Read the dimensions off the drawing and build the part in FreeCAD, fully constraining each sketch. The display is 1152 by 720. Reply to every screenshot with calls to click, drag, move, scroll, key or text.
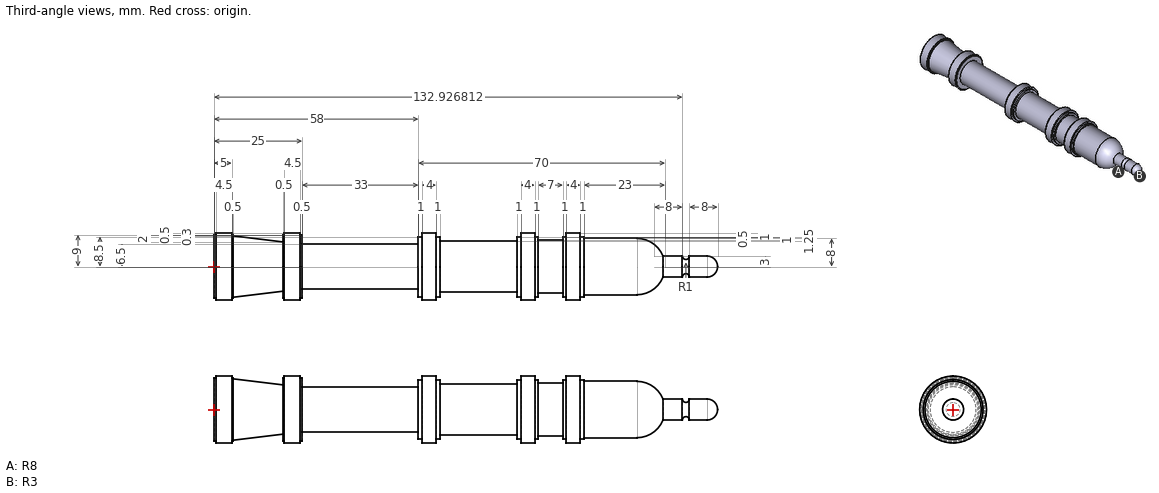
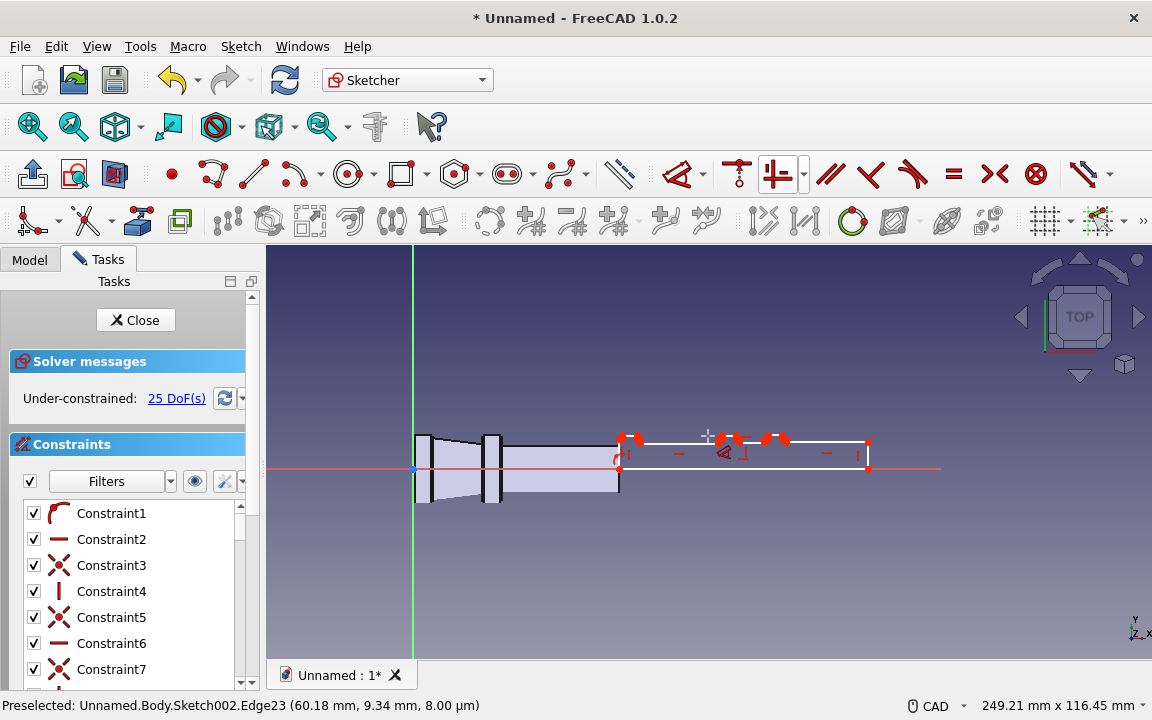
scroll(868, 461, up, 3)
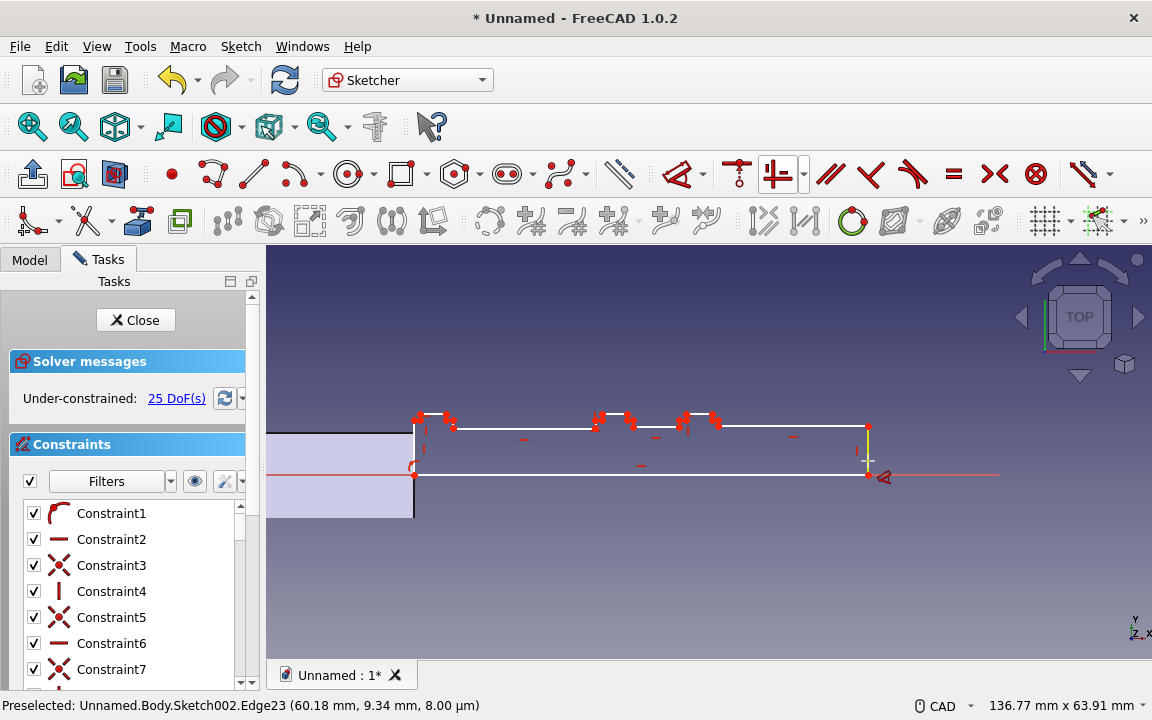
click(868, 461)
click(902, 451)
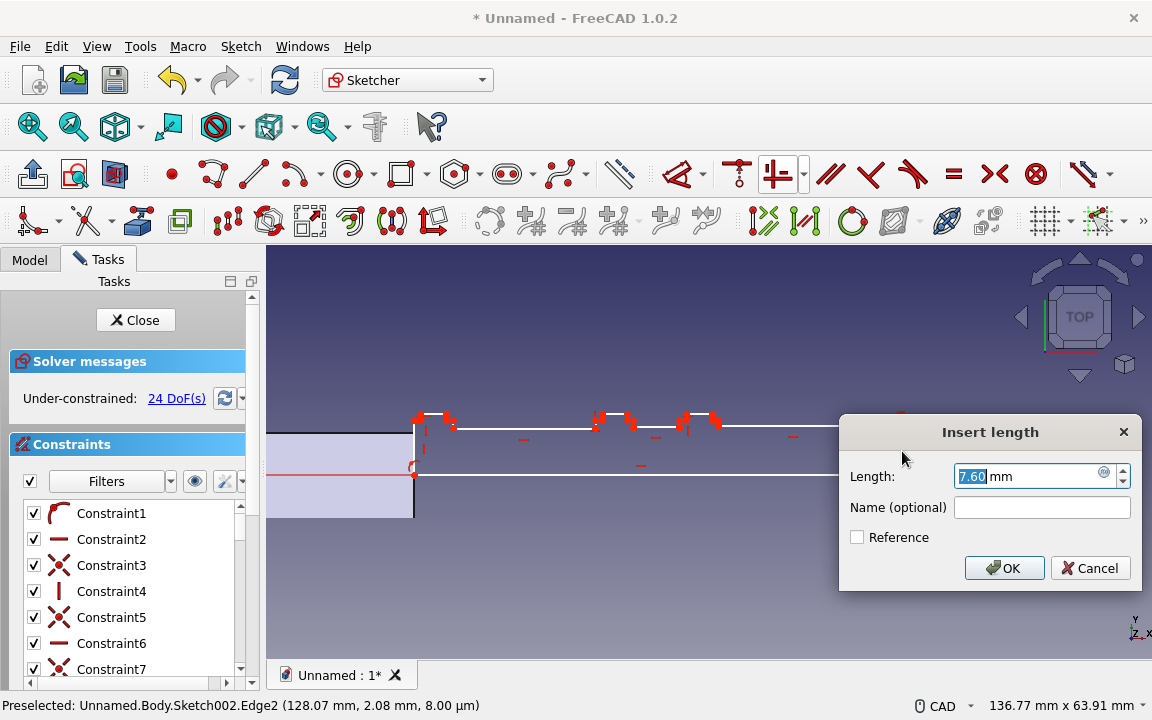
text(8)
key(Return)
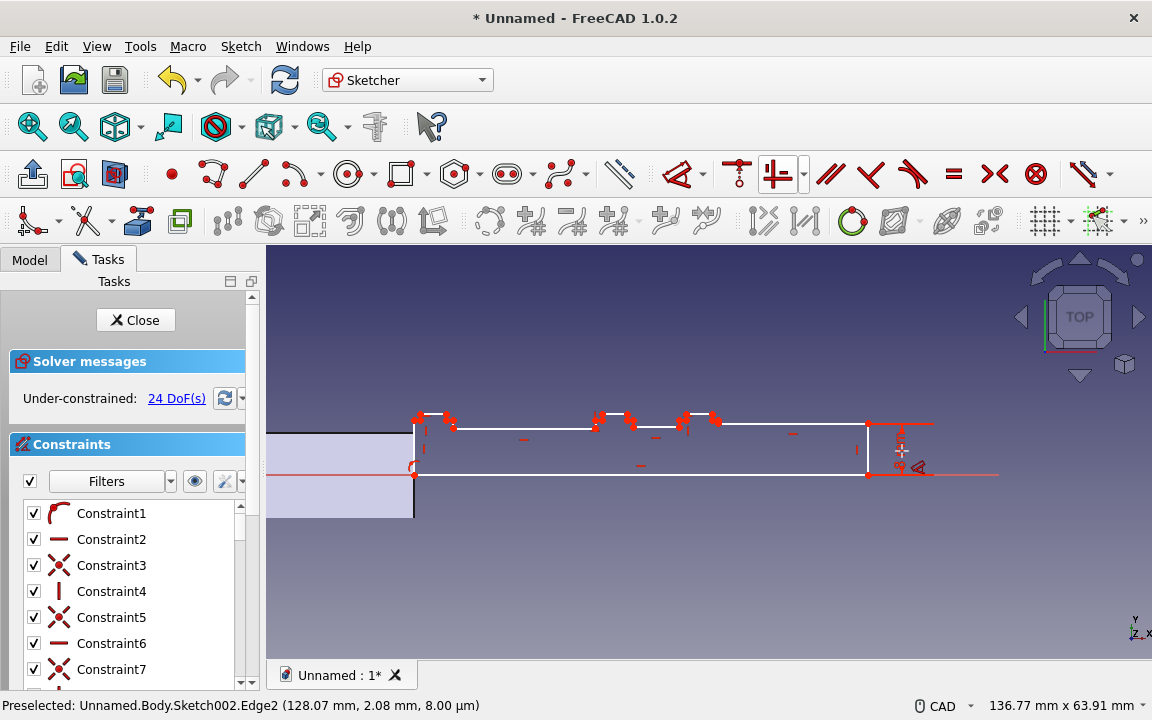
scroll(715, 421, up, 10)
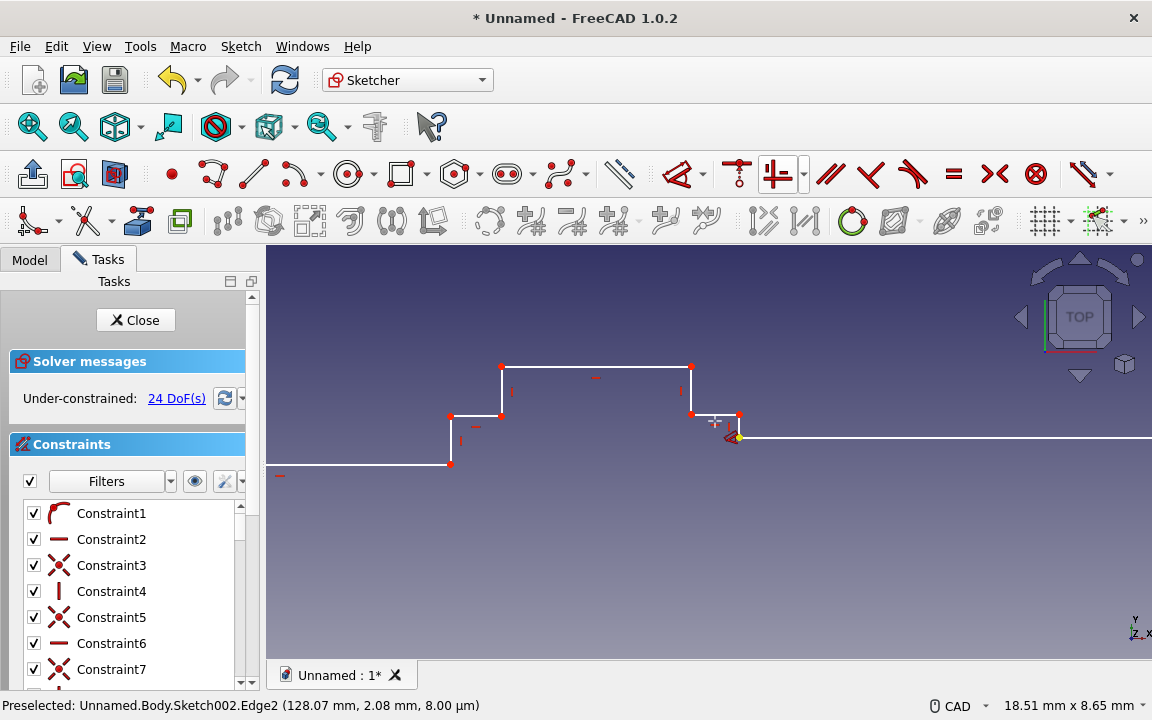
click(715, 415)
click(715, 381)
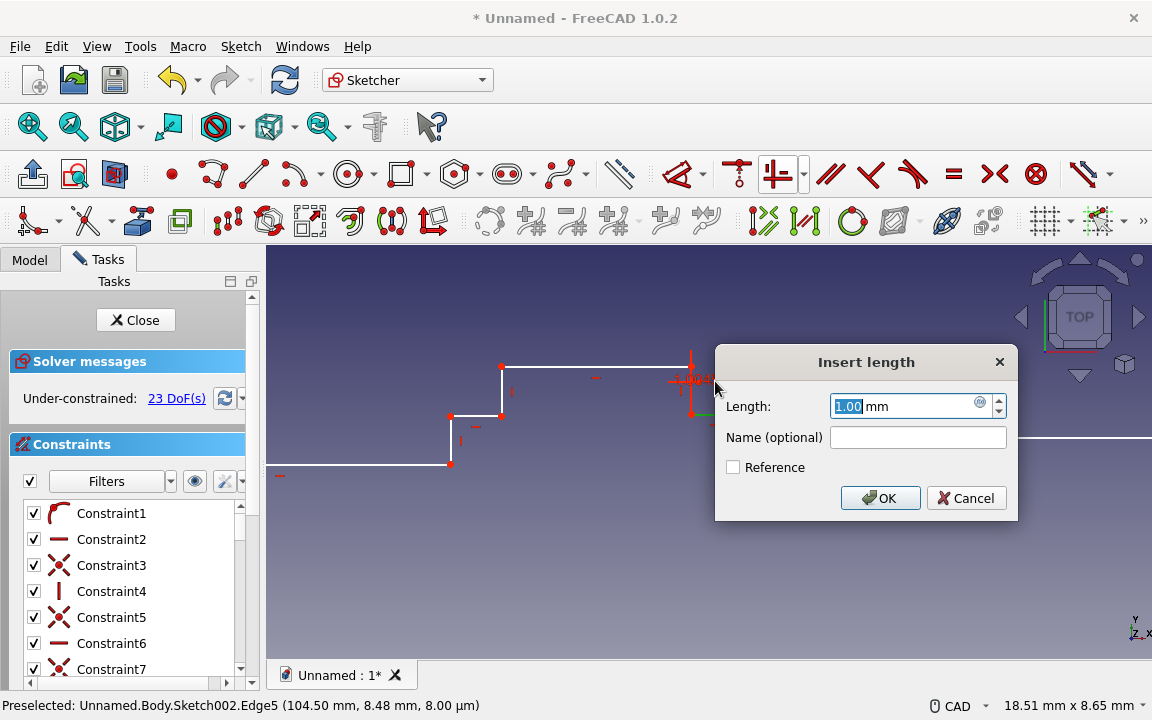
text(1)
key(Return)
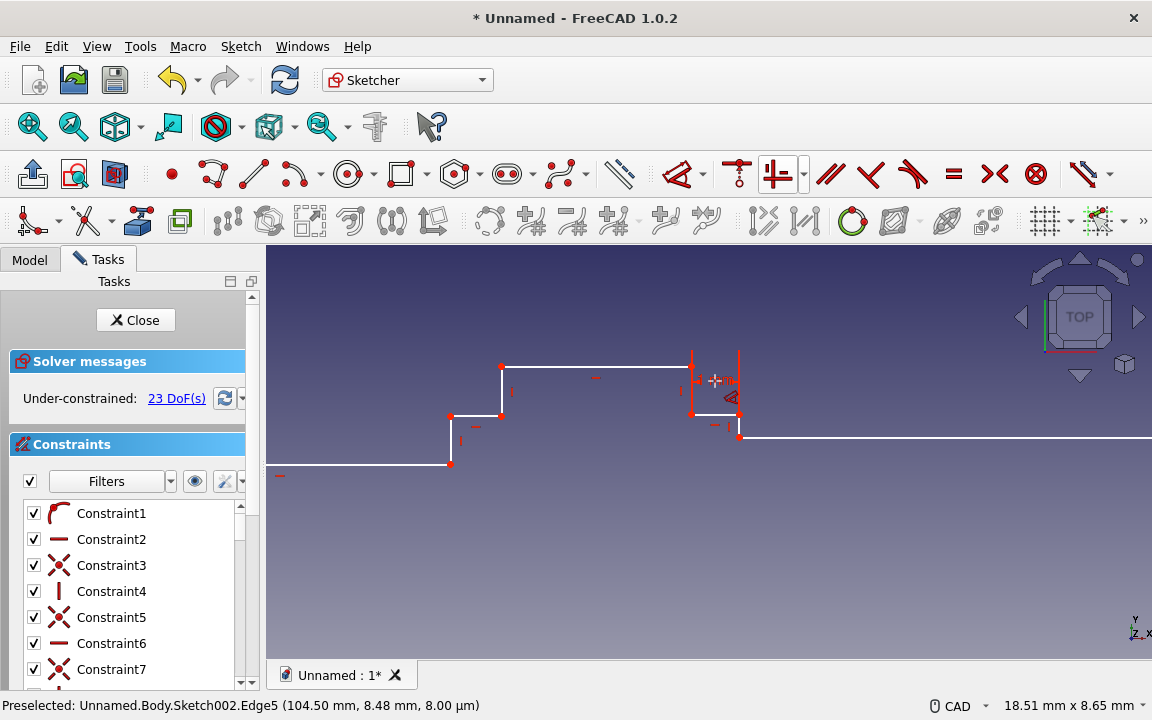
click(692, 400)
click(658, 402)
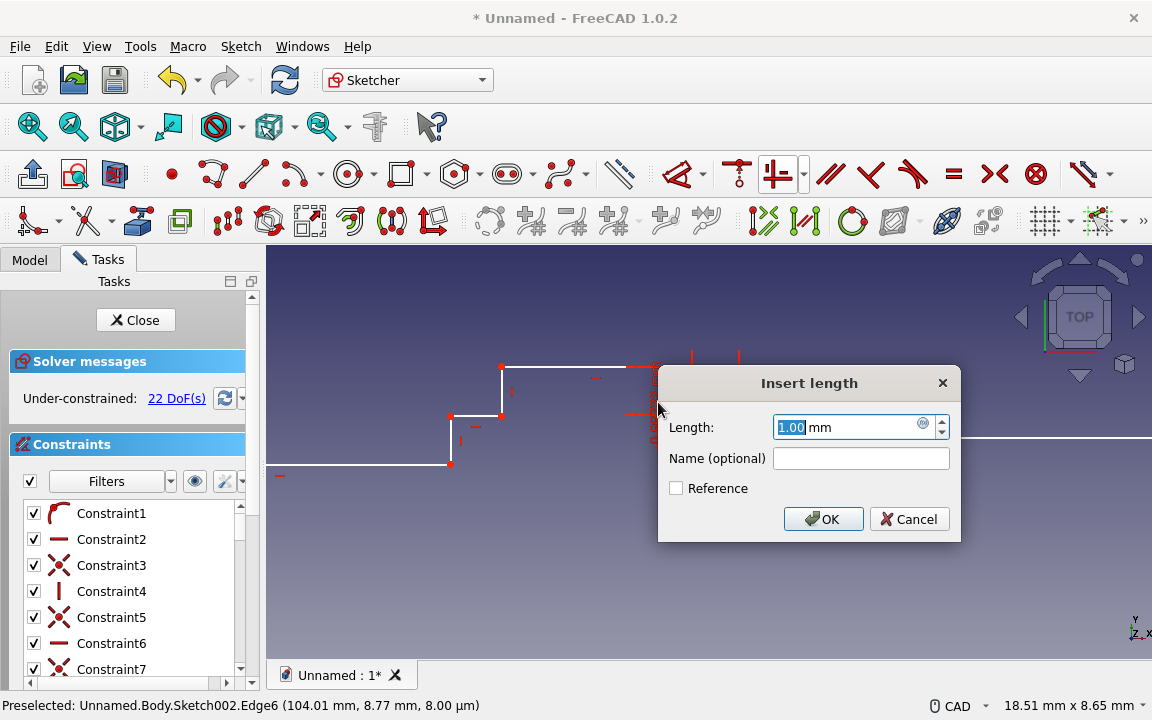
text(1)
key(Return)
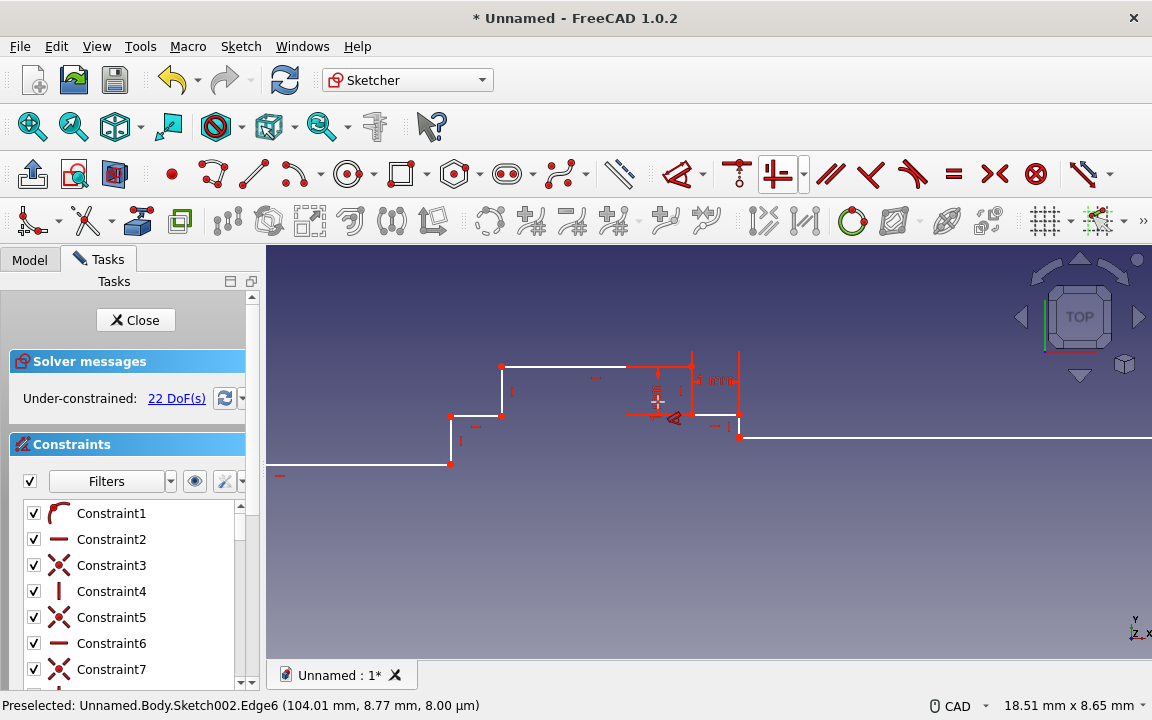
scroll(790, 441, down, 13)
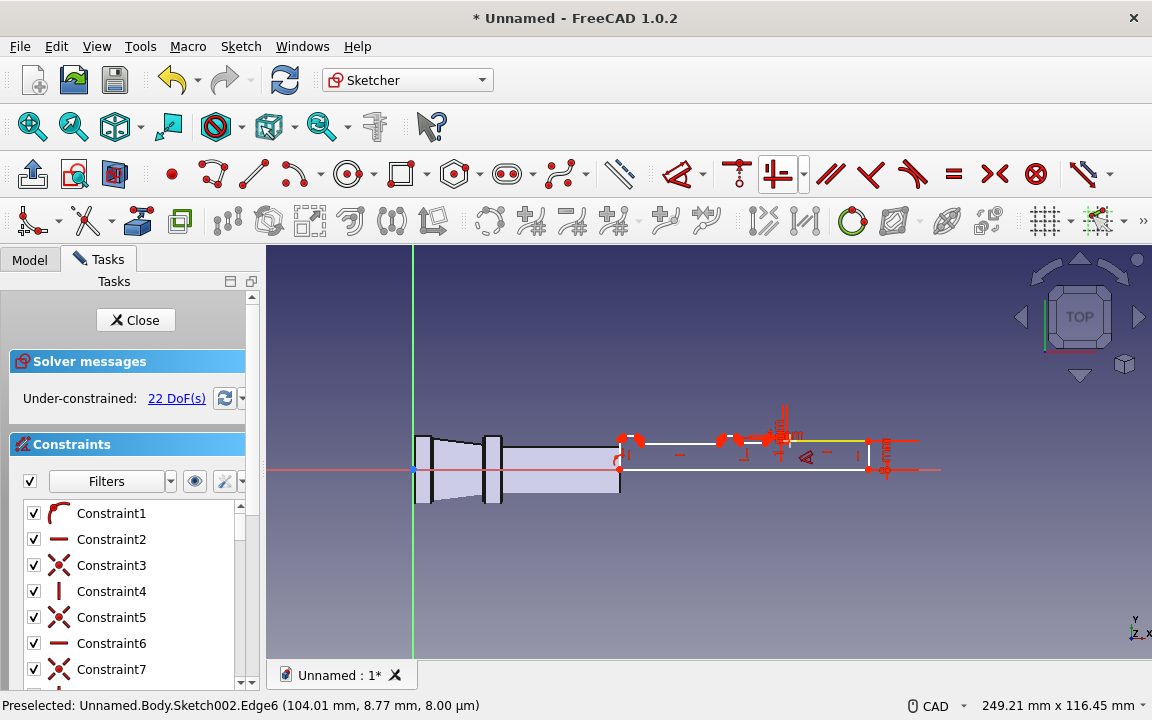
scroll(779, 436, up, 6)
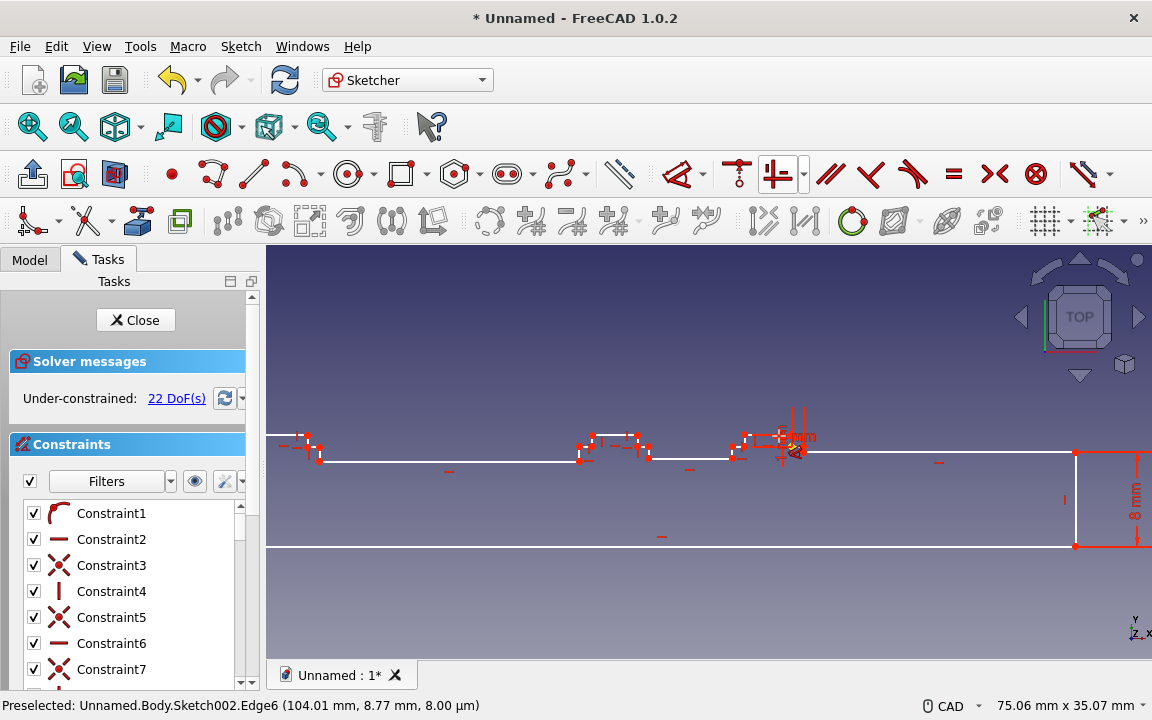
click(778, 435)
click(768, 401)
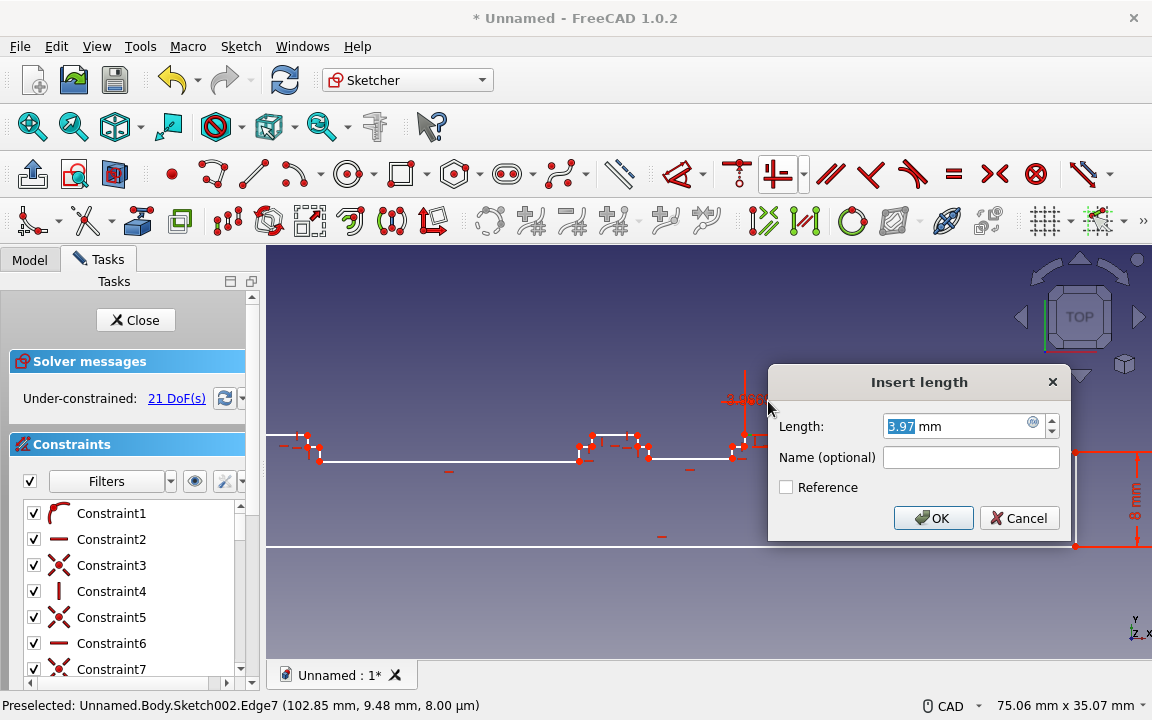
text(4)
key(Return)